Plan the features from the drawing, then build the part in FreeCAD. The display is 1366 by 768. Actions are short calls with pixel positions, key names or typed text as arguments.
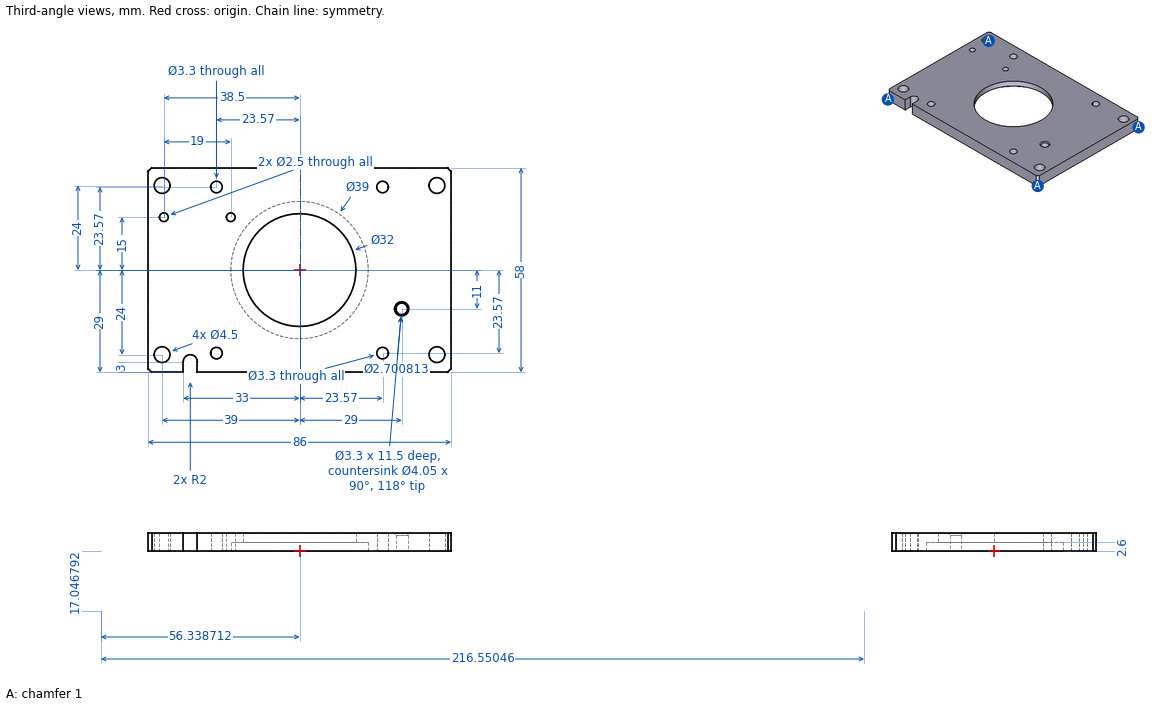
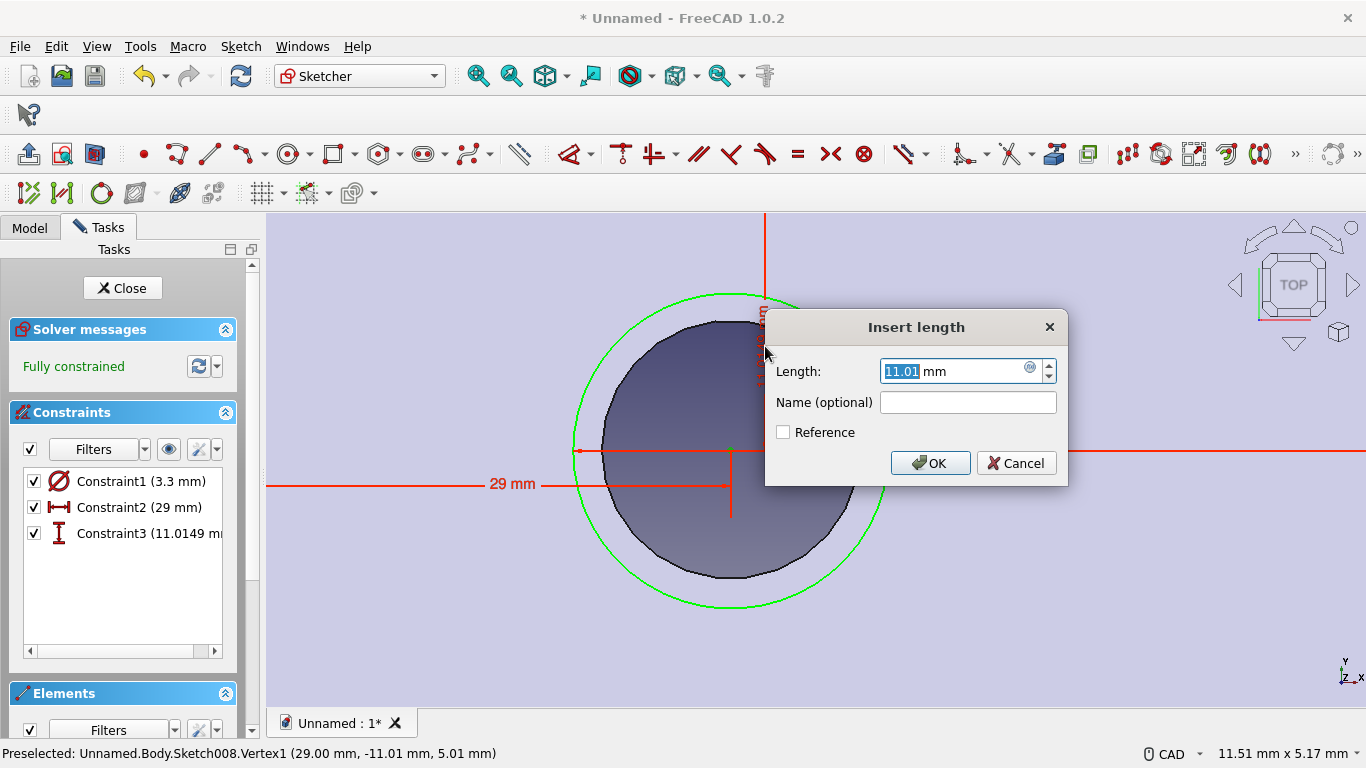
text(11)
key(Return)
key(Escape)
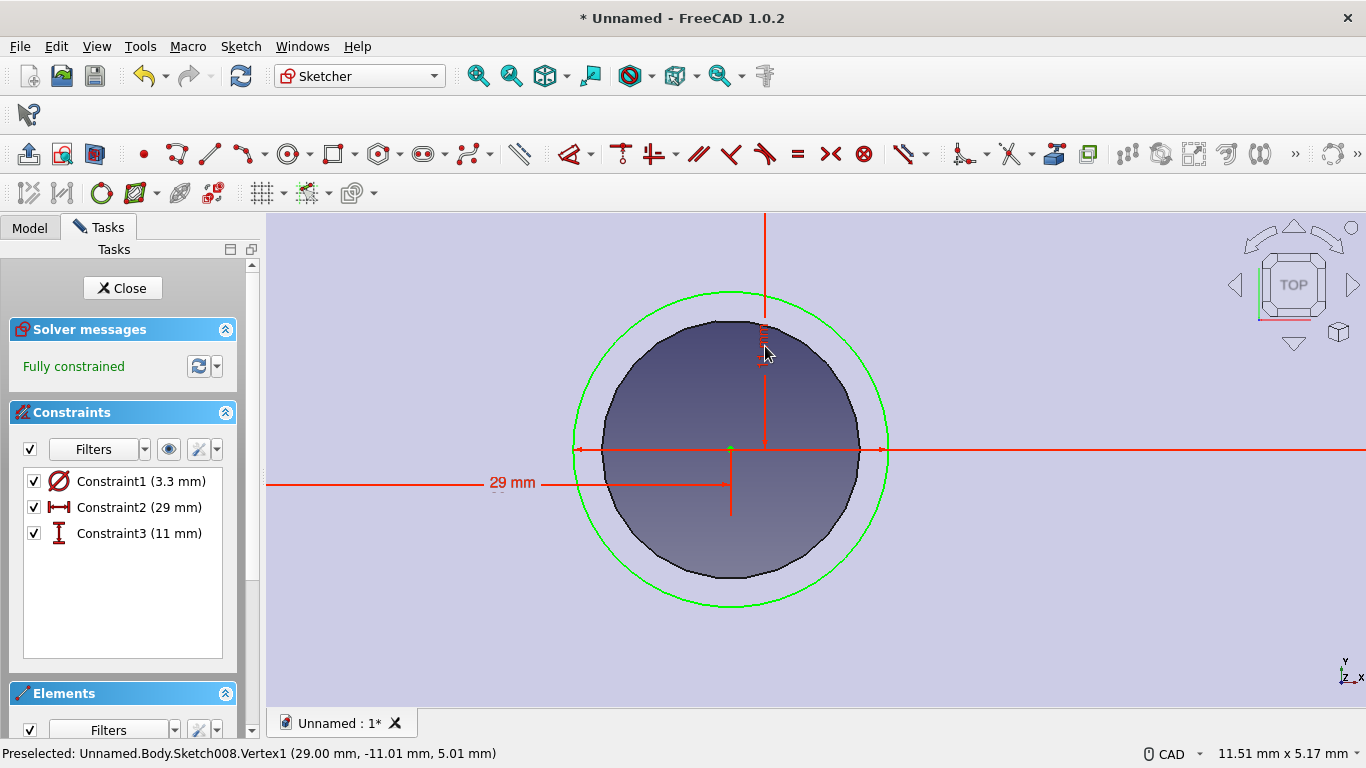
click(123, 288)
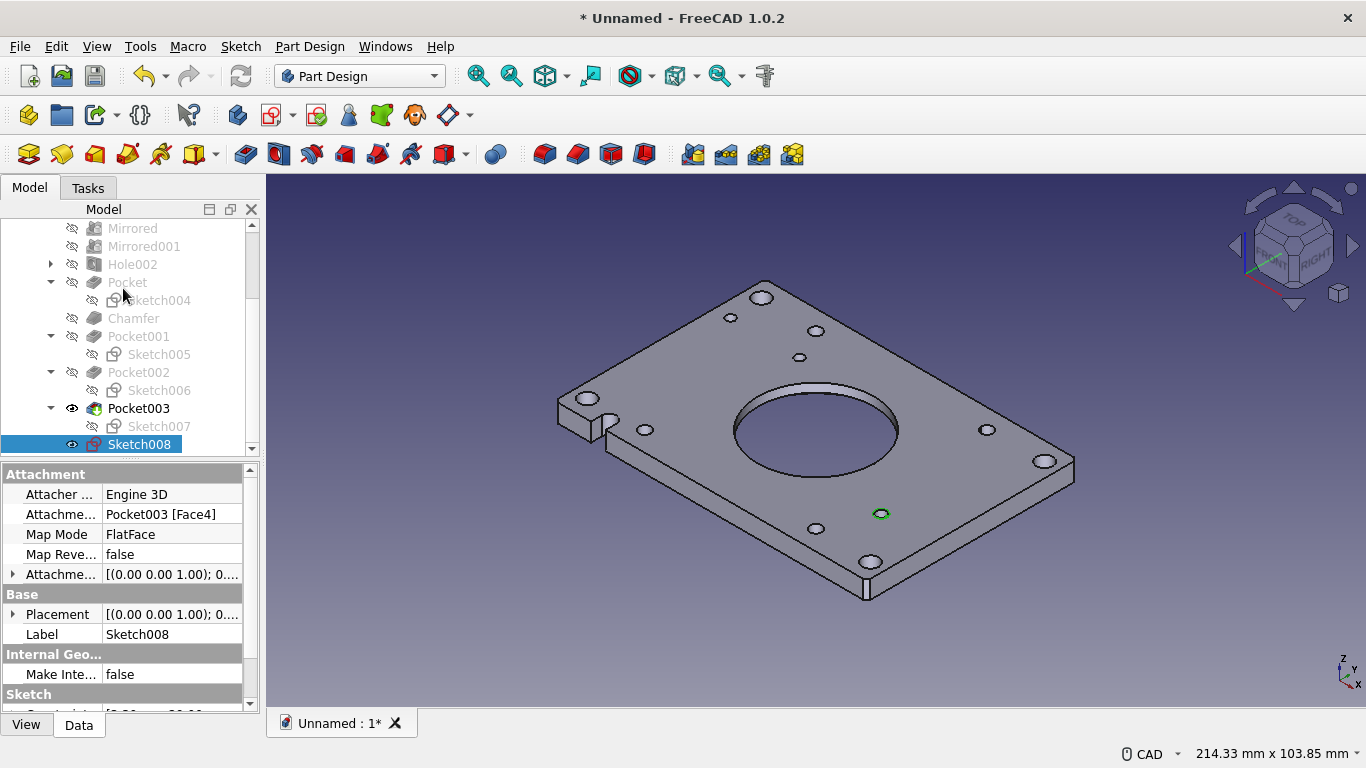
click(279, 154)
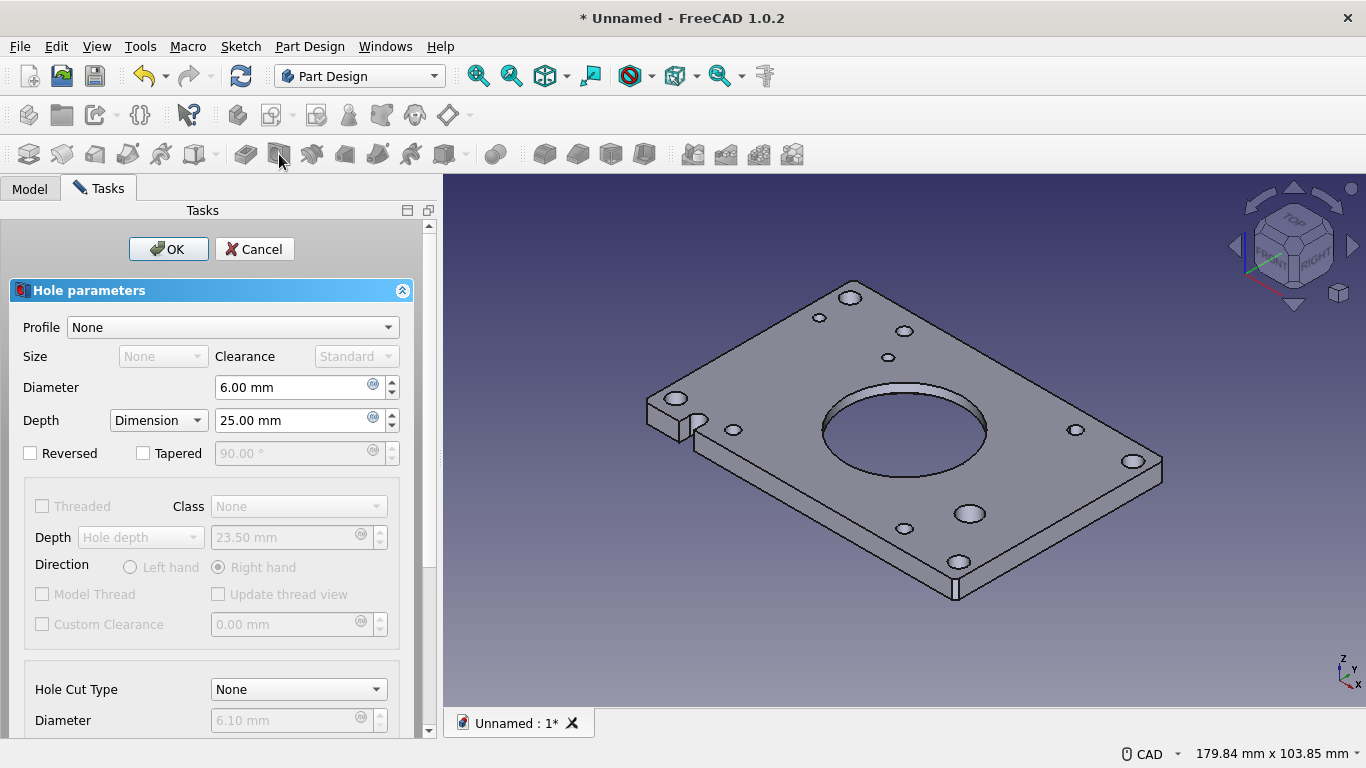
triple_click(300, 388)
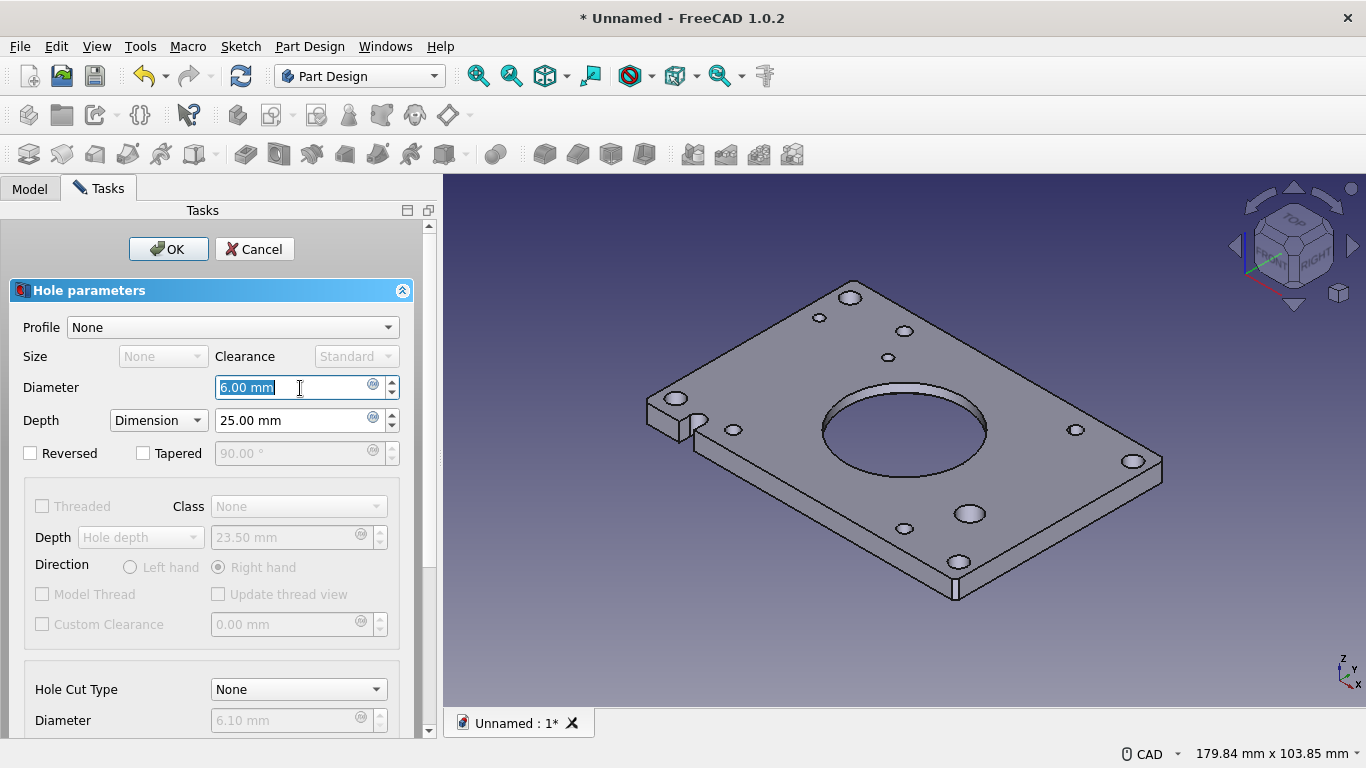
text(3.3)
key(Tab)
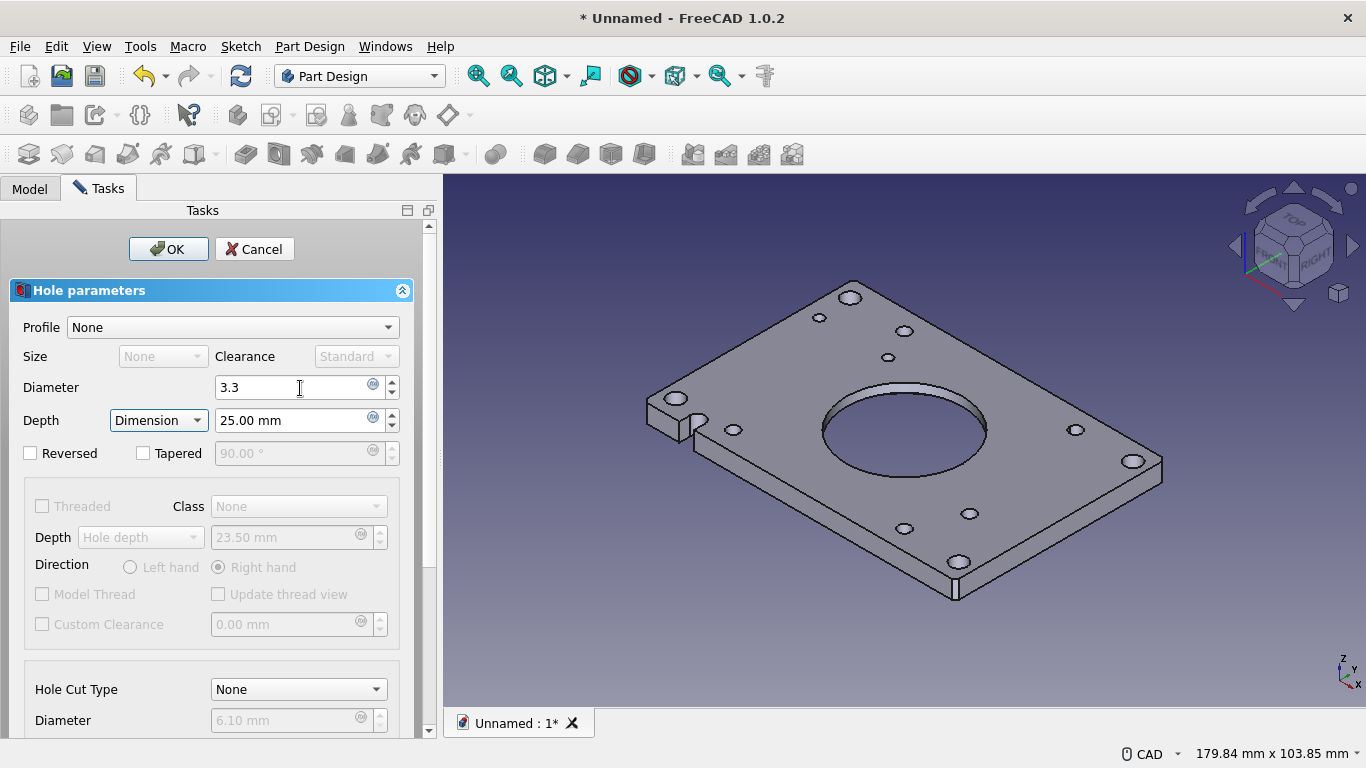
triple_click(300, 420)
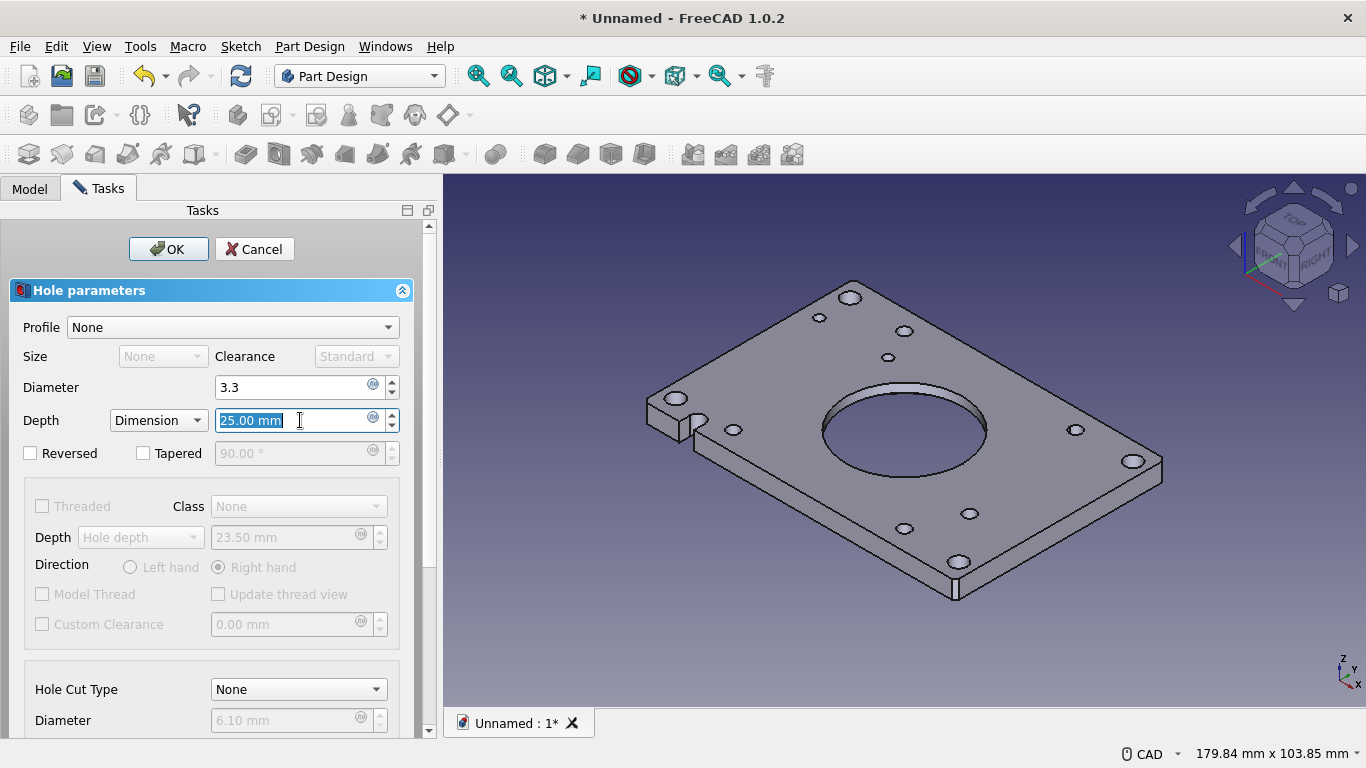
text(11.5)
key(Tab)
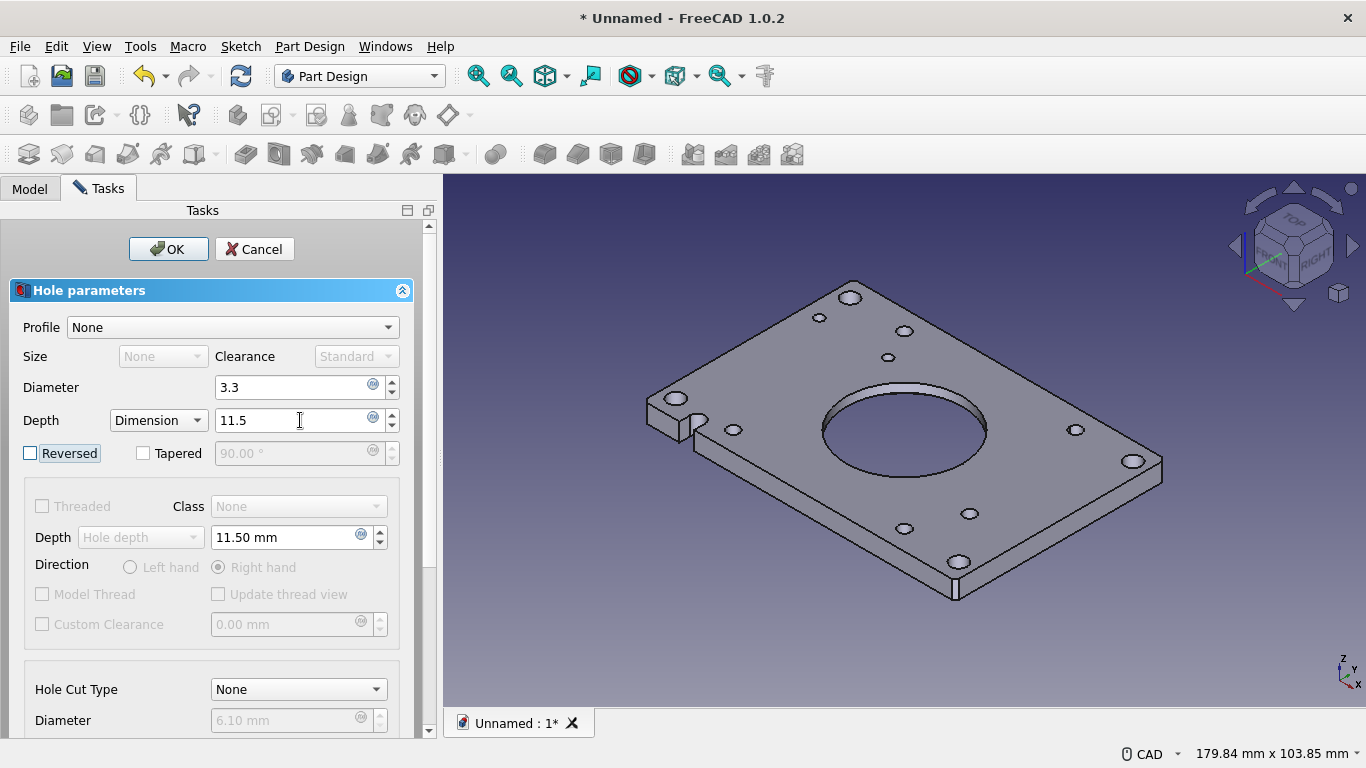
click(300, 690)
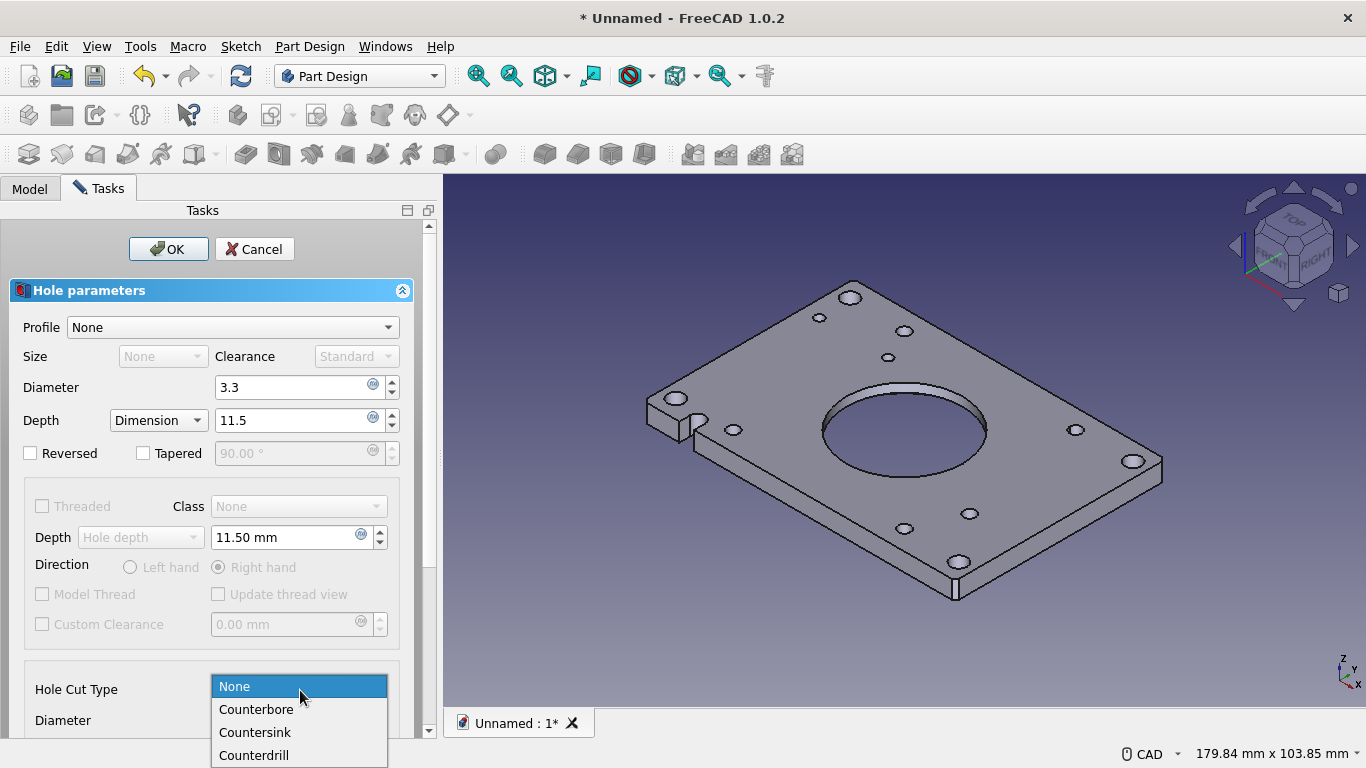
click(298, 732)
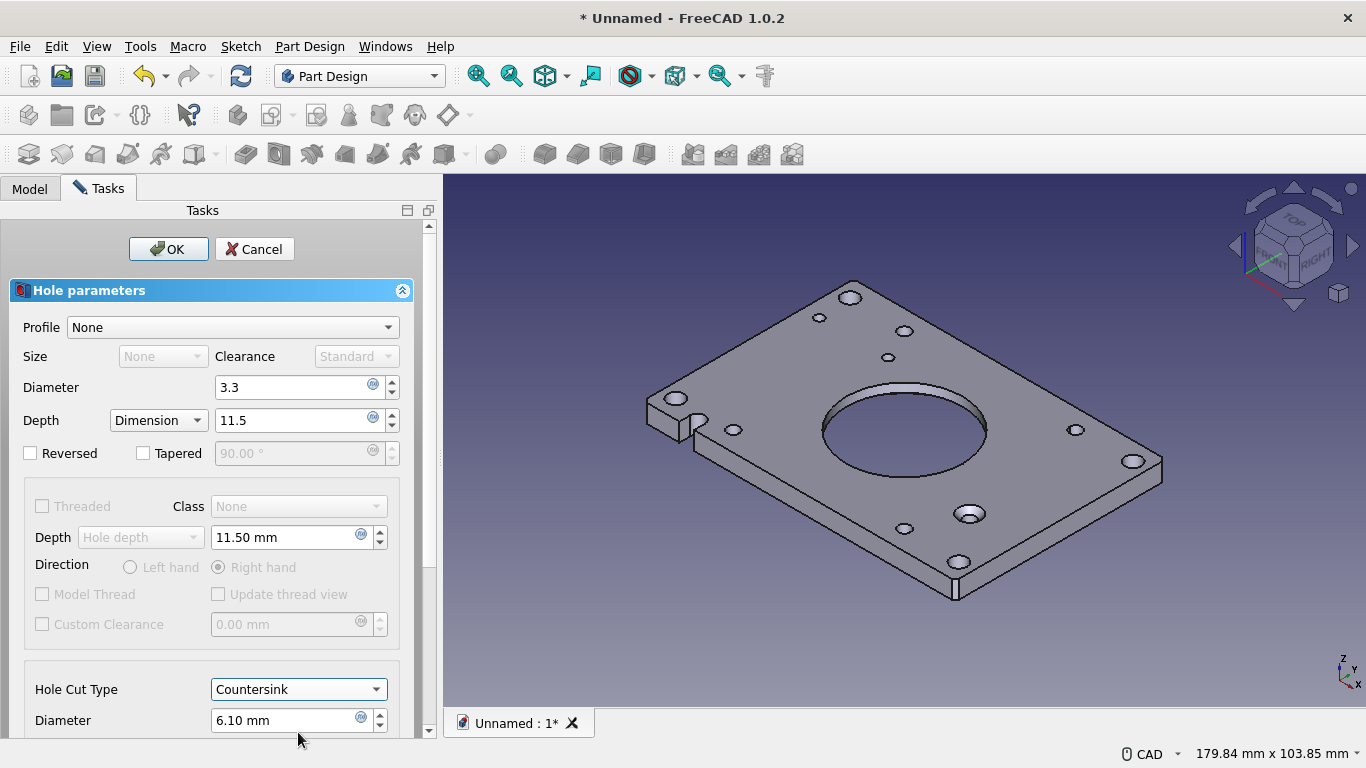
triple_click(292, 720)